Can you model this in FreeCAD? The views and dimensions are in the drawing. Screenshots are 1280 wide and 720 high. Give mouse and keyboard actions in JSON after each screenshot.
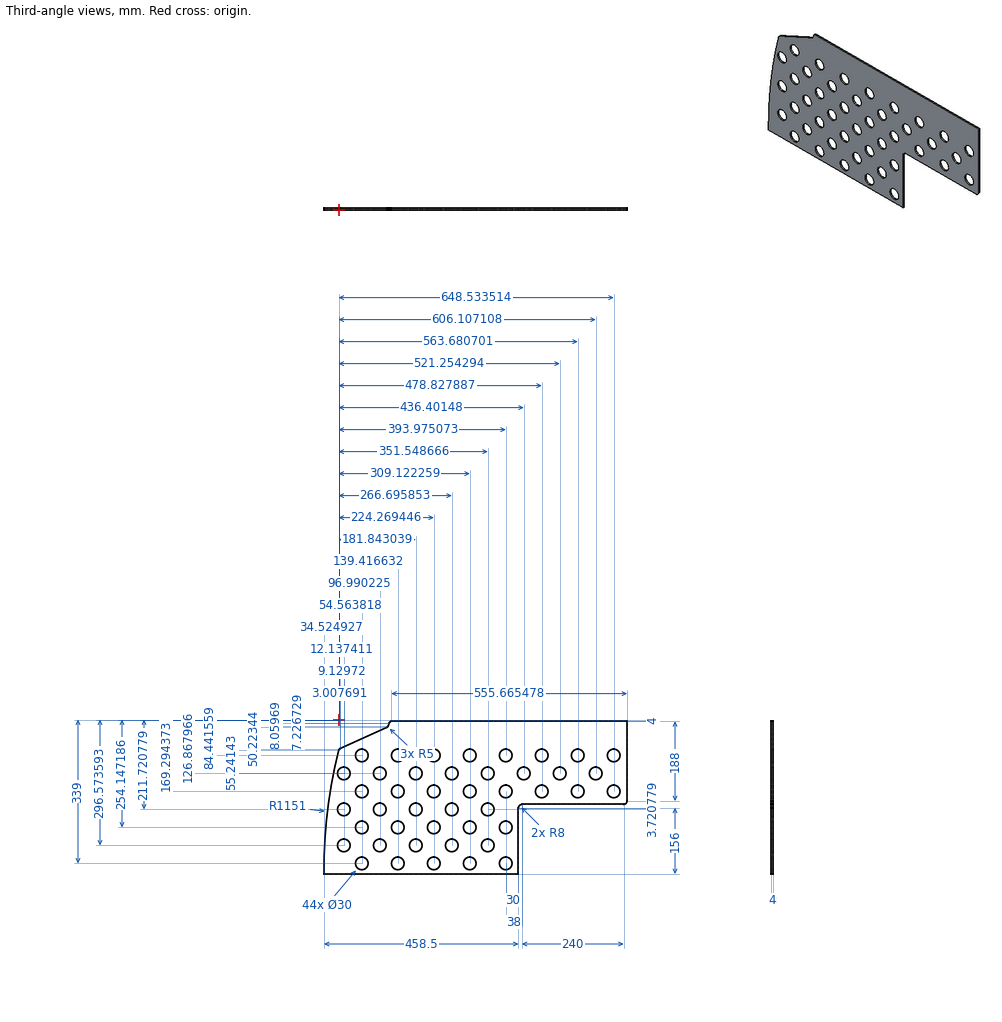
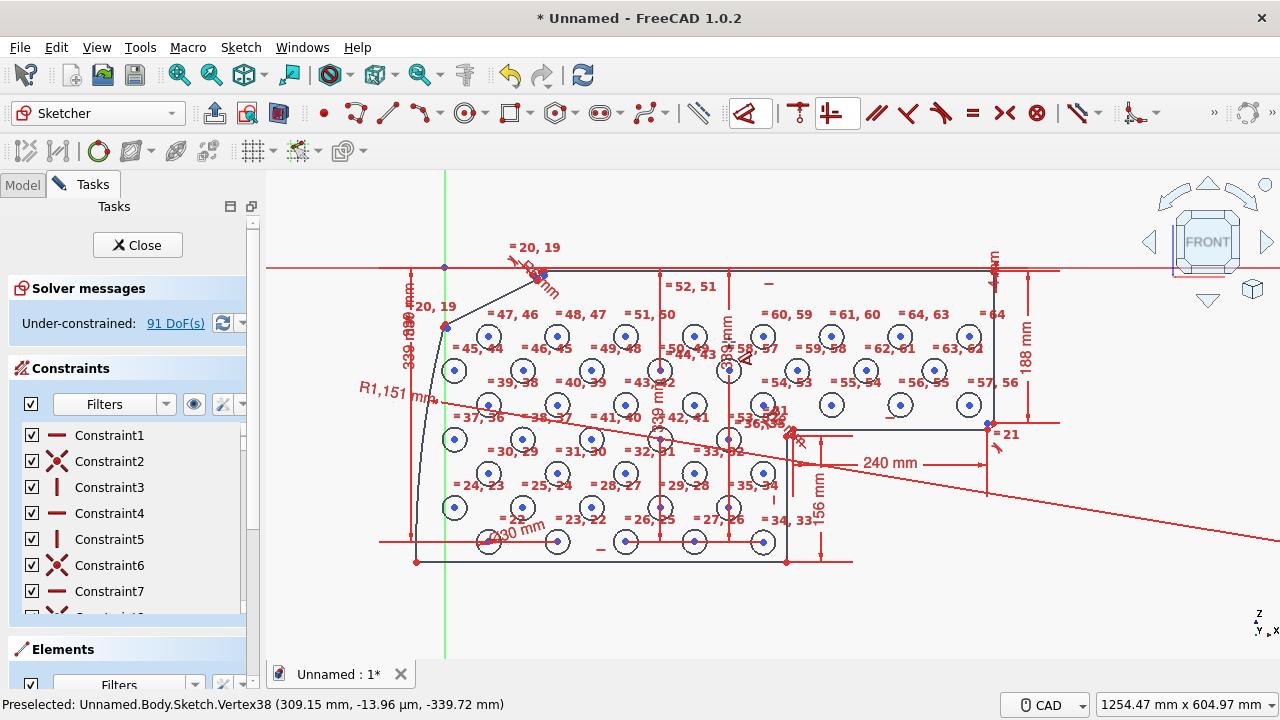
{"action": "left_click", "coordinate": [763, 543]}
{"action": "left_click", "coordinate": [797, 405]}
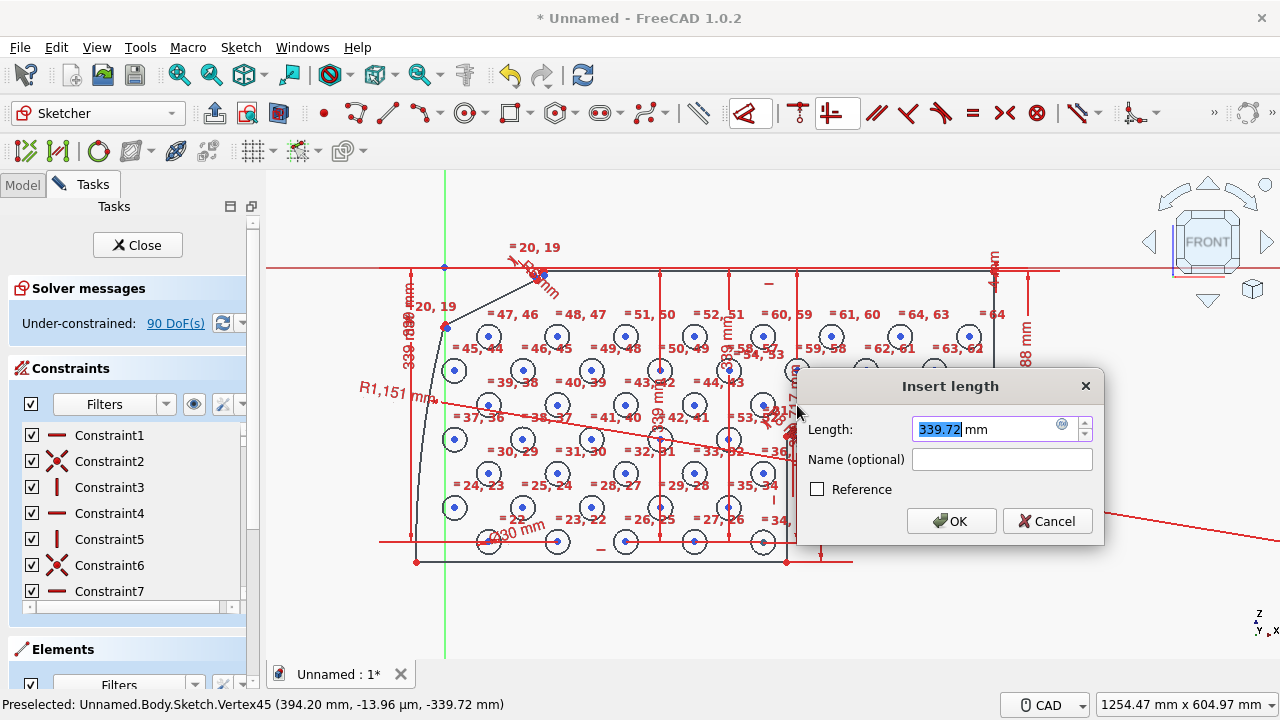
{"action": "type", "text": "339"}
{"action": "key", "text": "Return"}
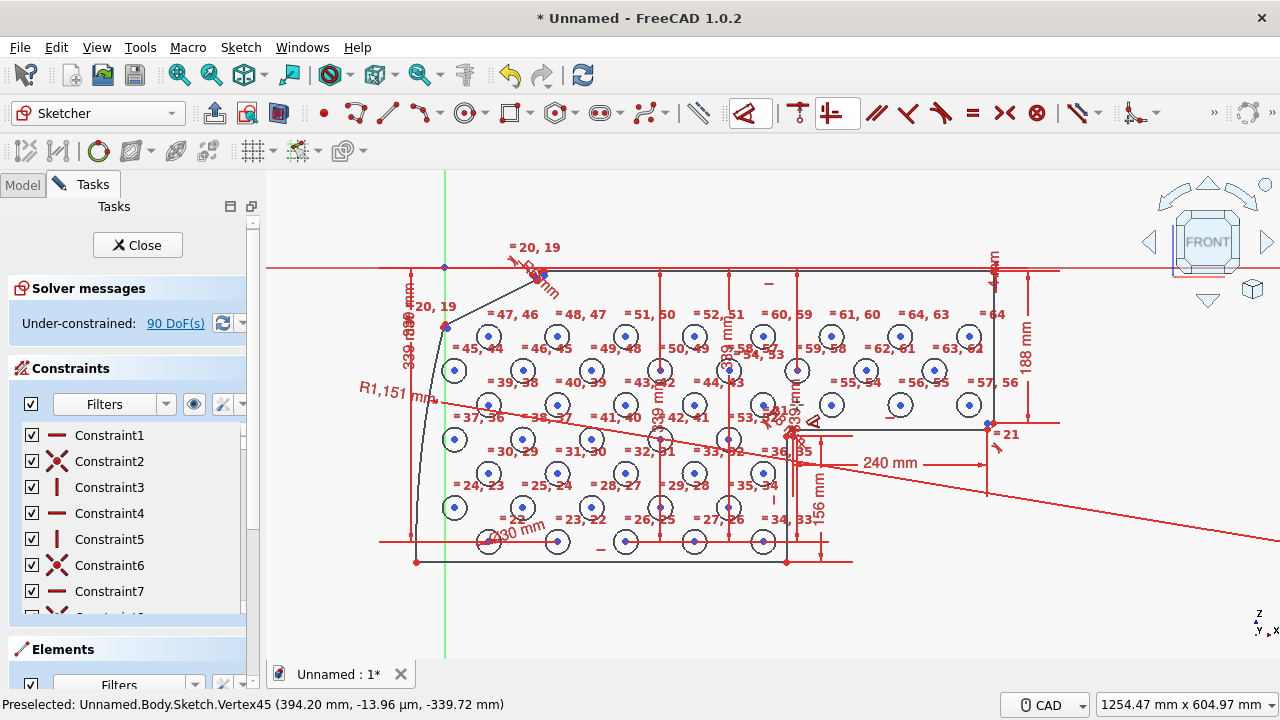
{"action": "scroll", "coordinate": [787, 562], "scroll_direction": "up", "scroll_amount": 3}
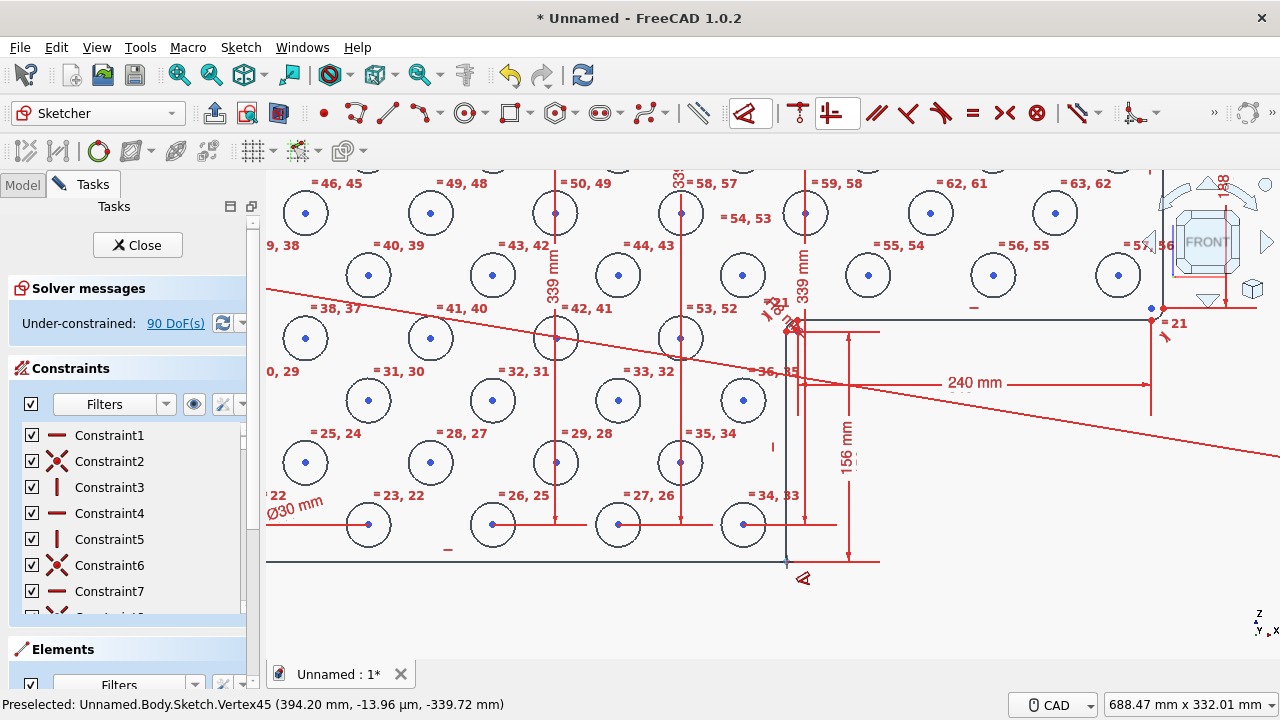
{"action": "left_click", "coordinate": [786, 562]}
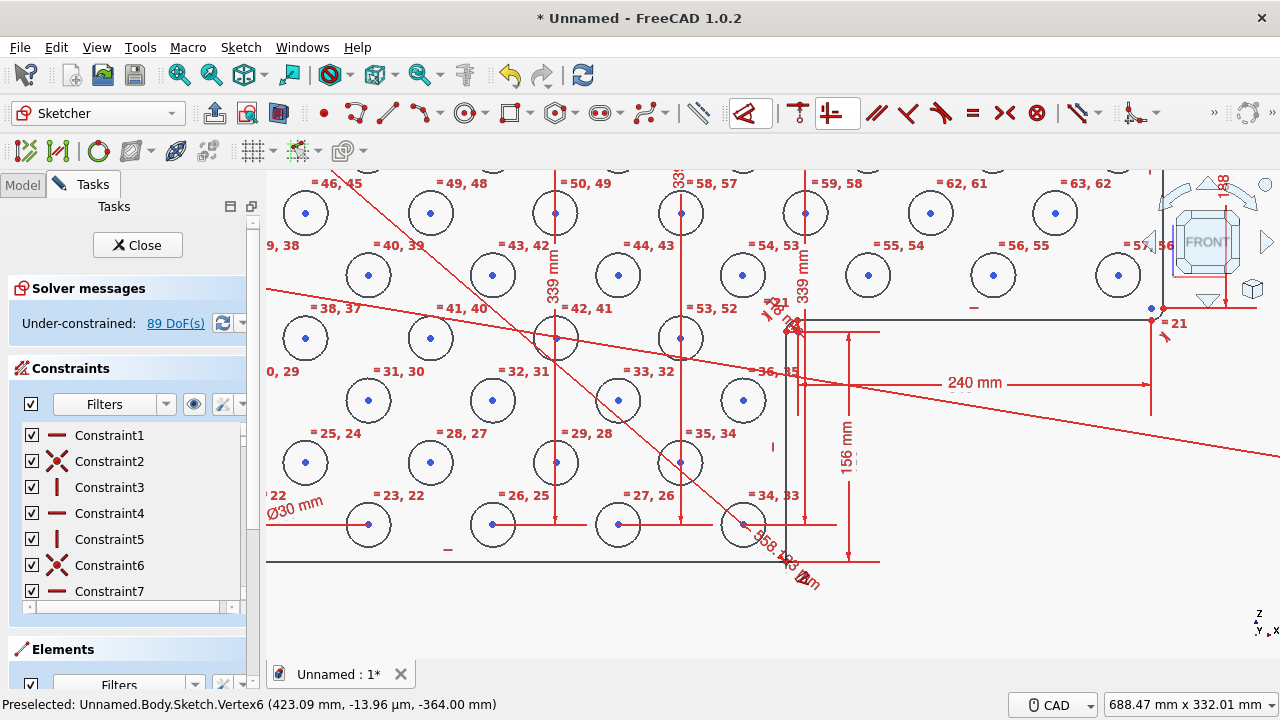
{"action": "left_click", "coordinate": [744, 525]}
{"action": "left_click", "coordinate": [765, 596]}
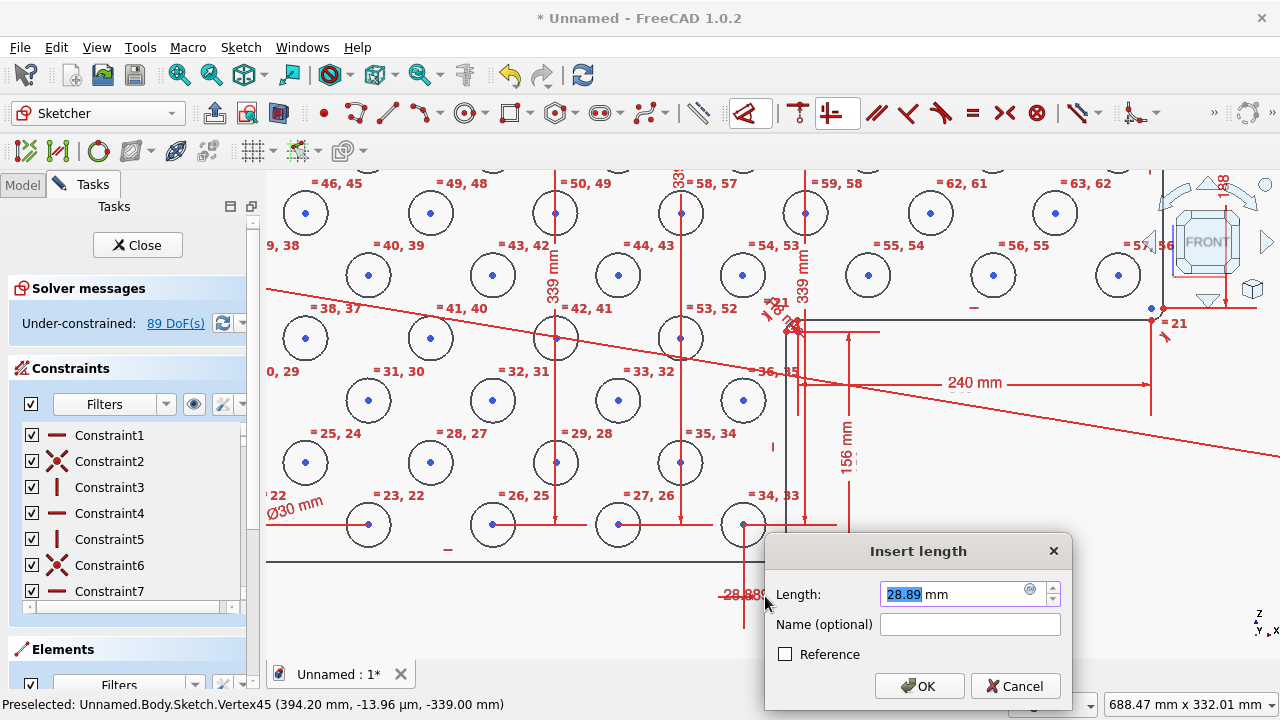
{"action": "type", "text": "30"}
{"action": "key", "text": "Return"}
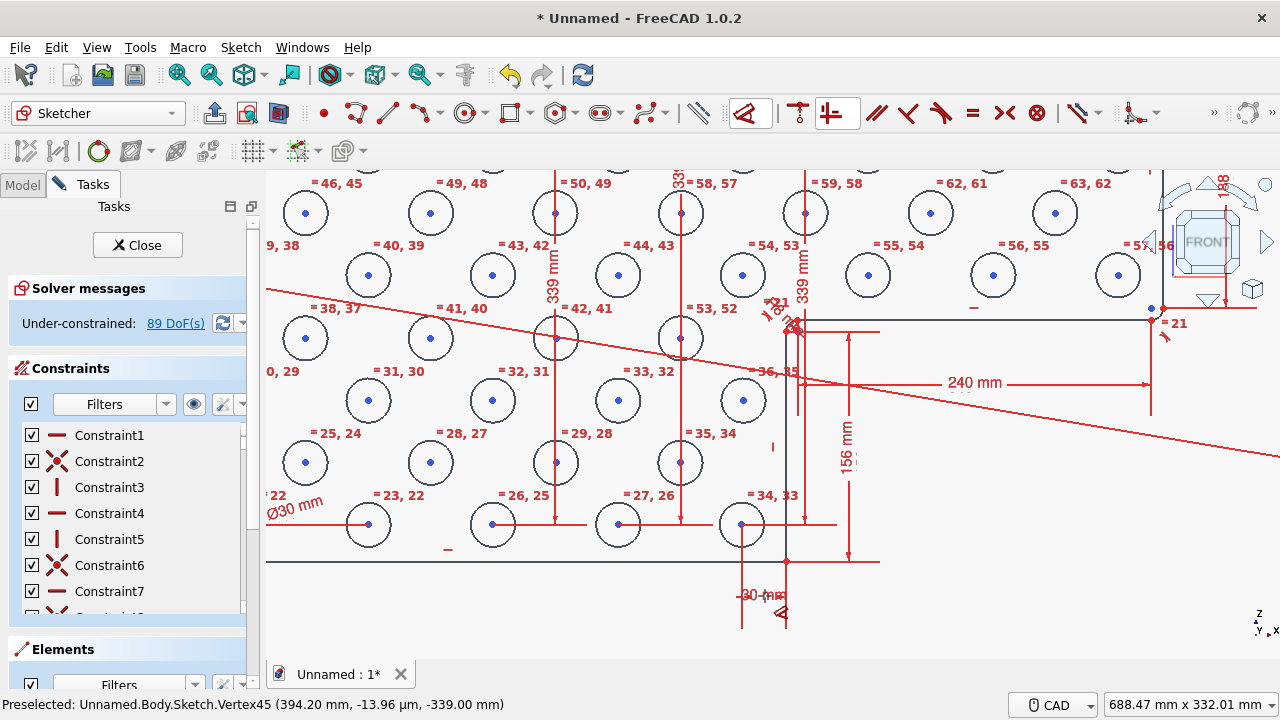
{"action": "left_click", "coordinate": [786, 332]}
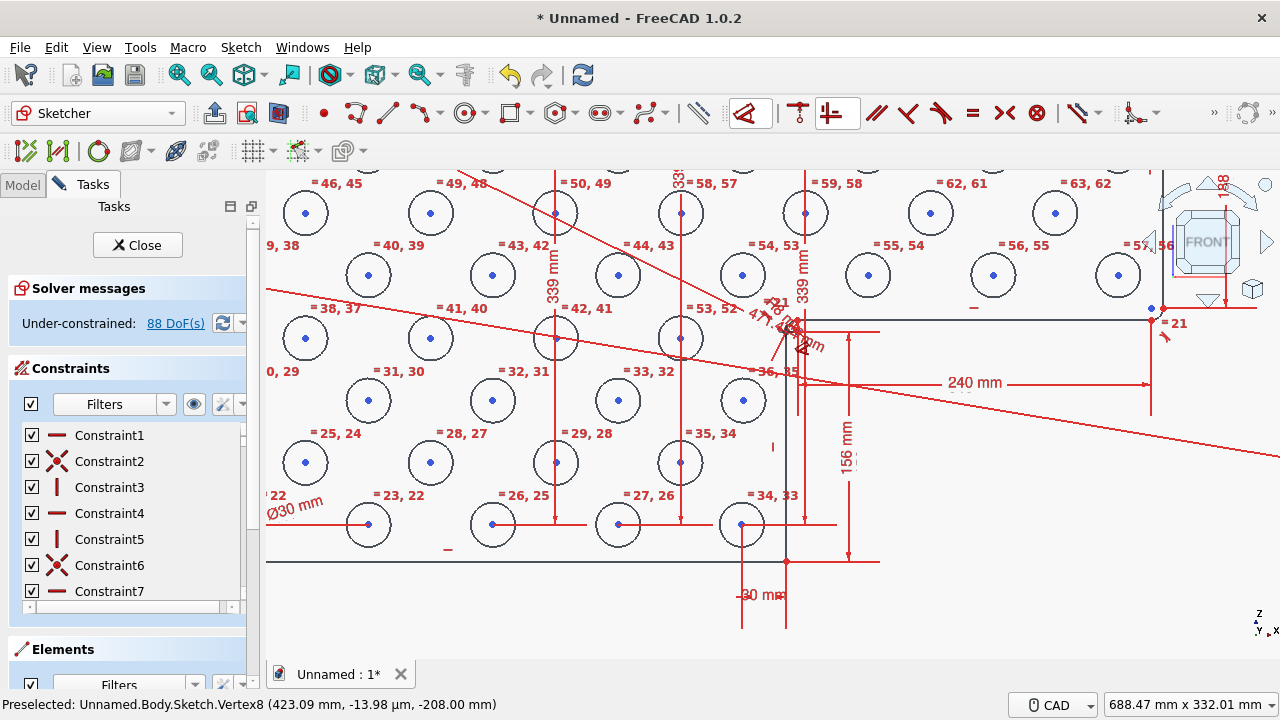
{"action": "left_click", "coordinate": [744, 401]}
{"action": "left_click", "coordinate": [765, 435]}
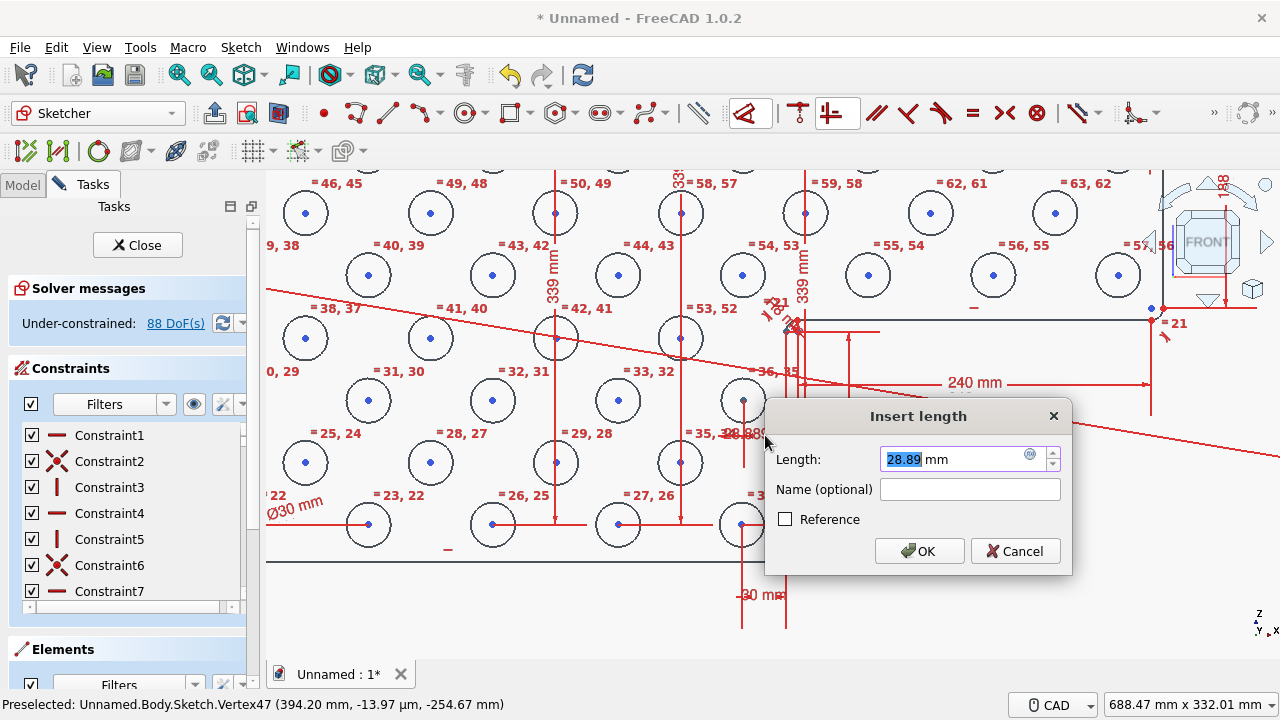
{"action": "type", "text": "30"}
{"action": "key", "text": "Return"}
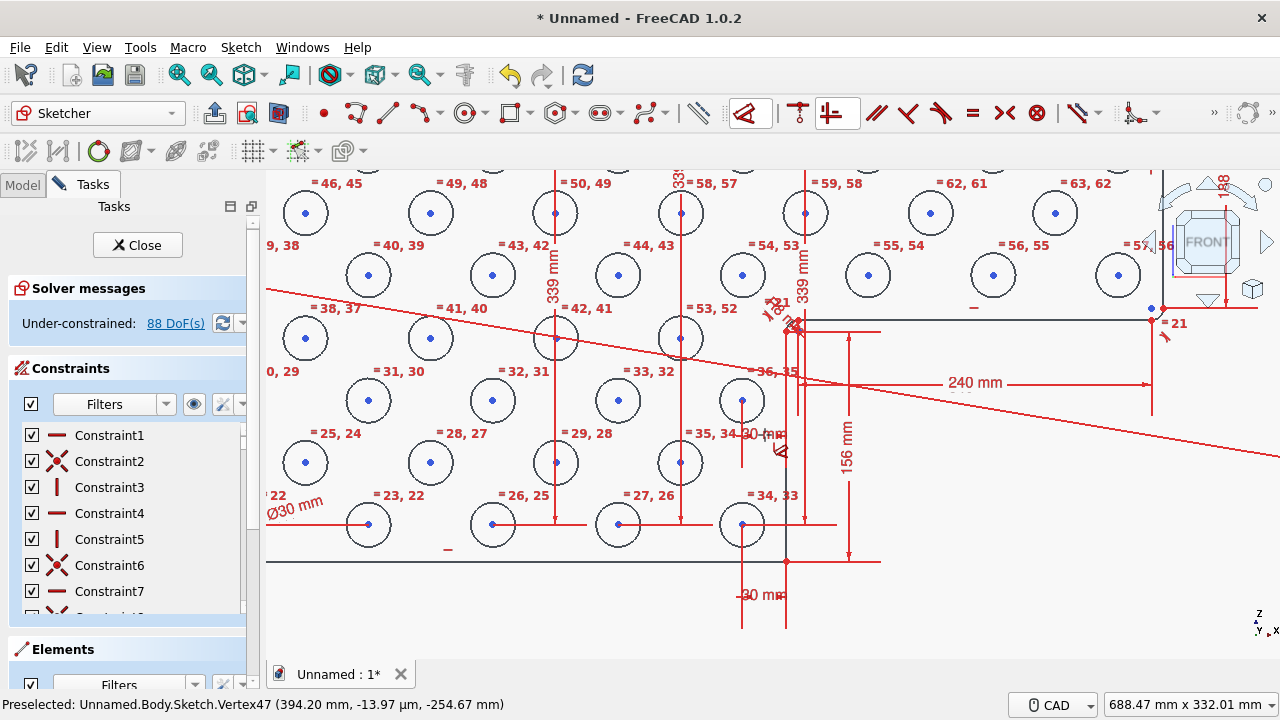
{"action": "left_click", "coordinate": [798, 320]}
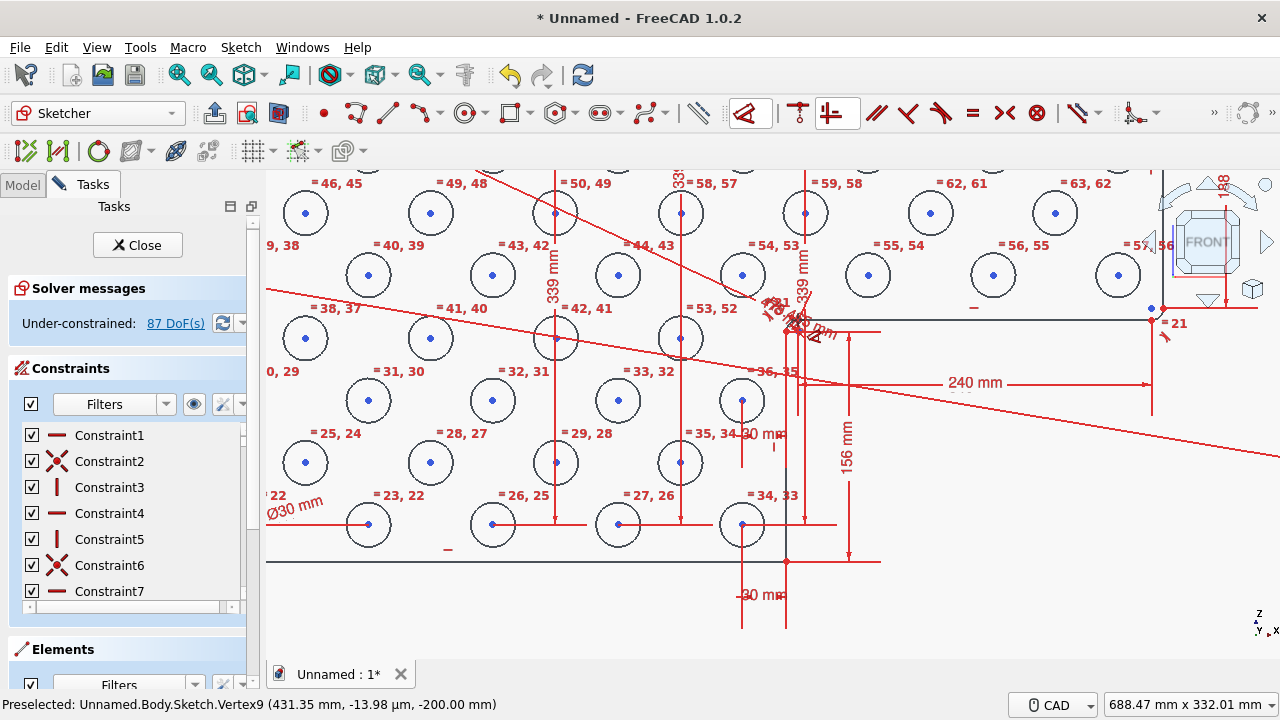
{"action": "left_click", "coordinate": [743, 275]}
{"action": "left_click", "coordinate": [771, 354]}